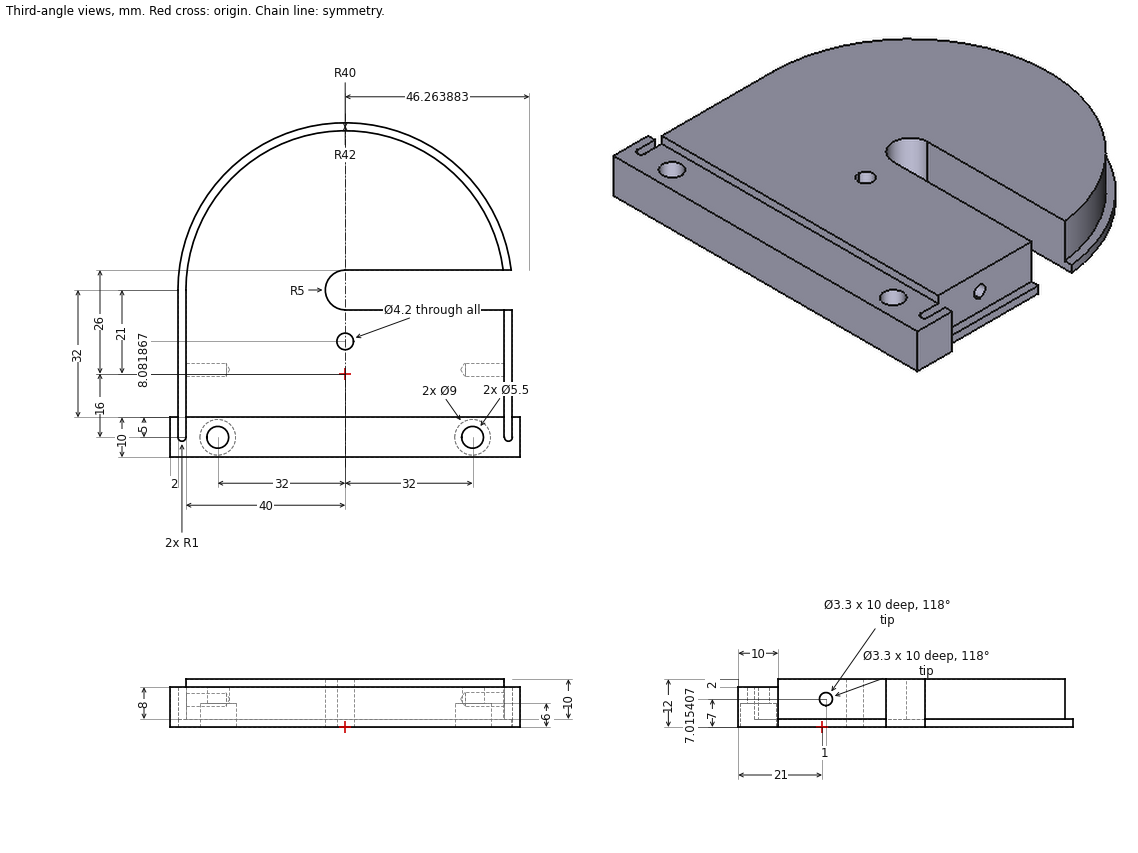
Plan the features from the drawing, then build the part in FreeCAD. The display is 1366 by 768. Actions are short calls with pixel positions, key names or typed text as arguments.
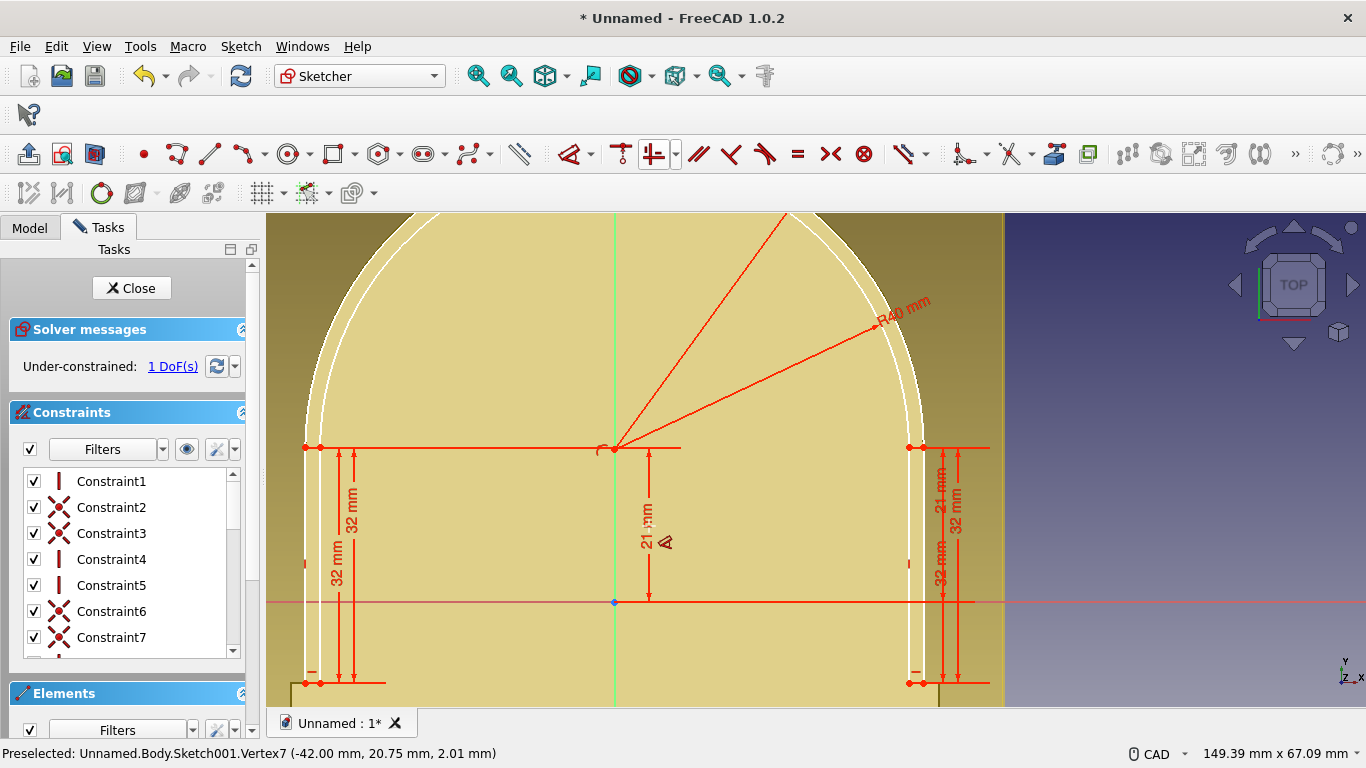
click(615, 450)
click(649, 491)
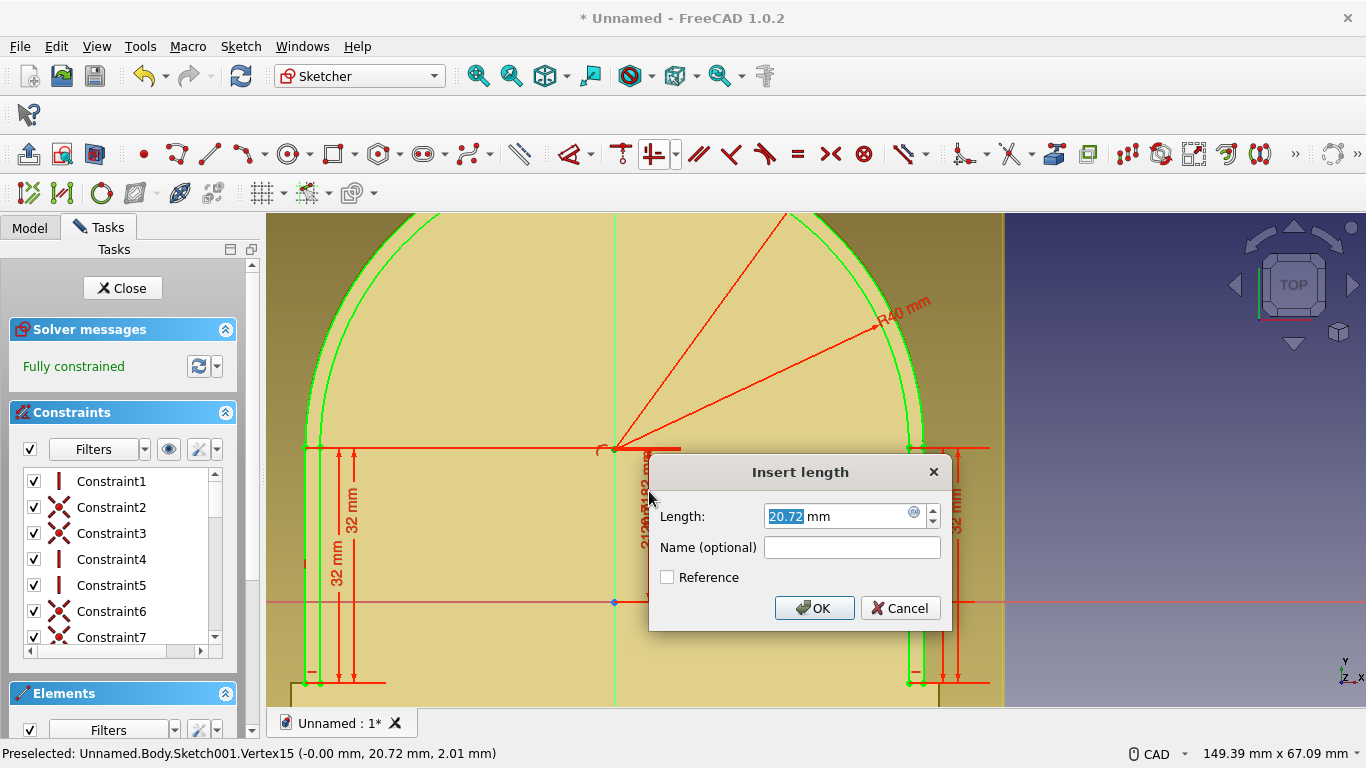
text(21)
key(Return)
key(Escape)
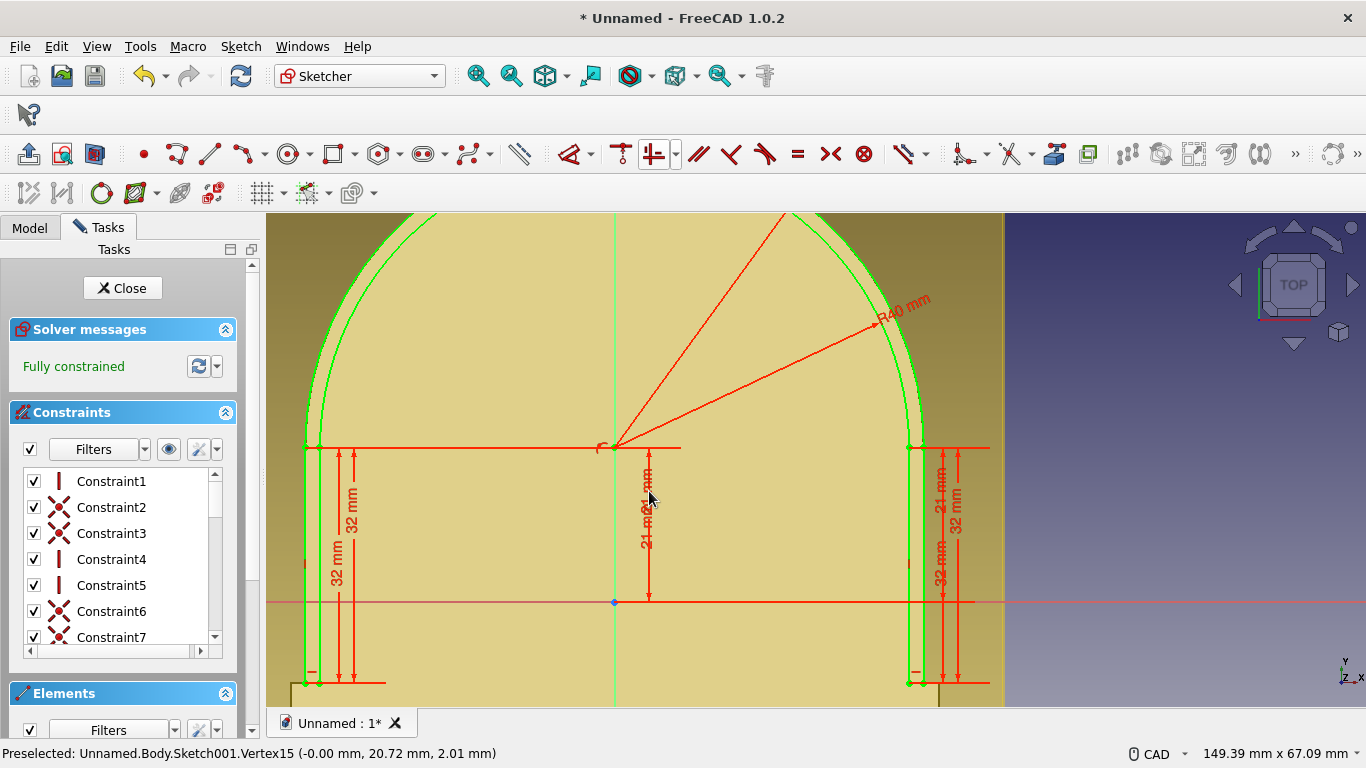
click(123, 288)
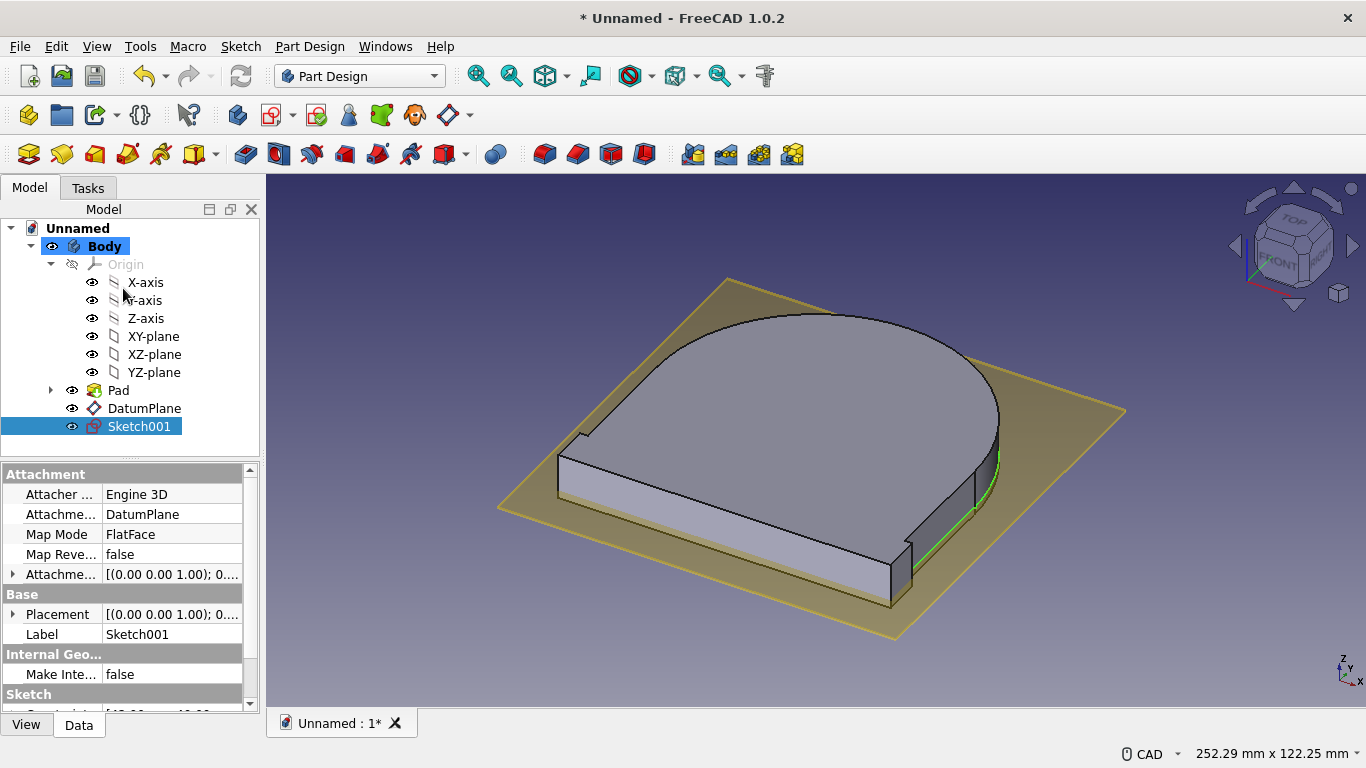
click(246, 154)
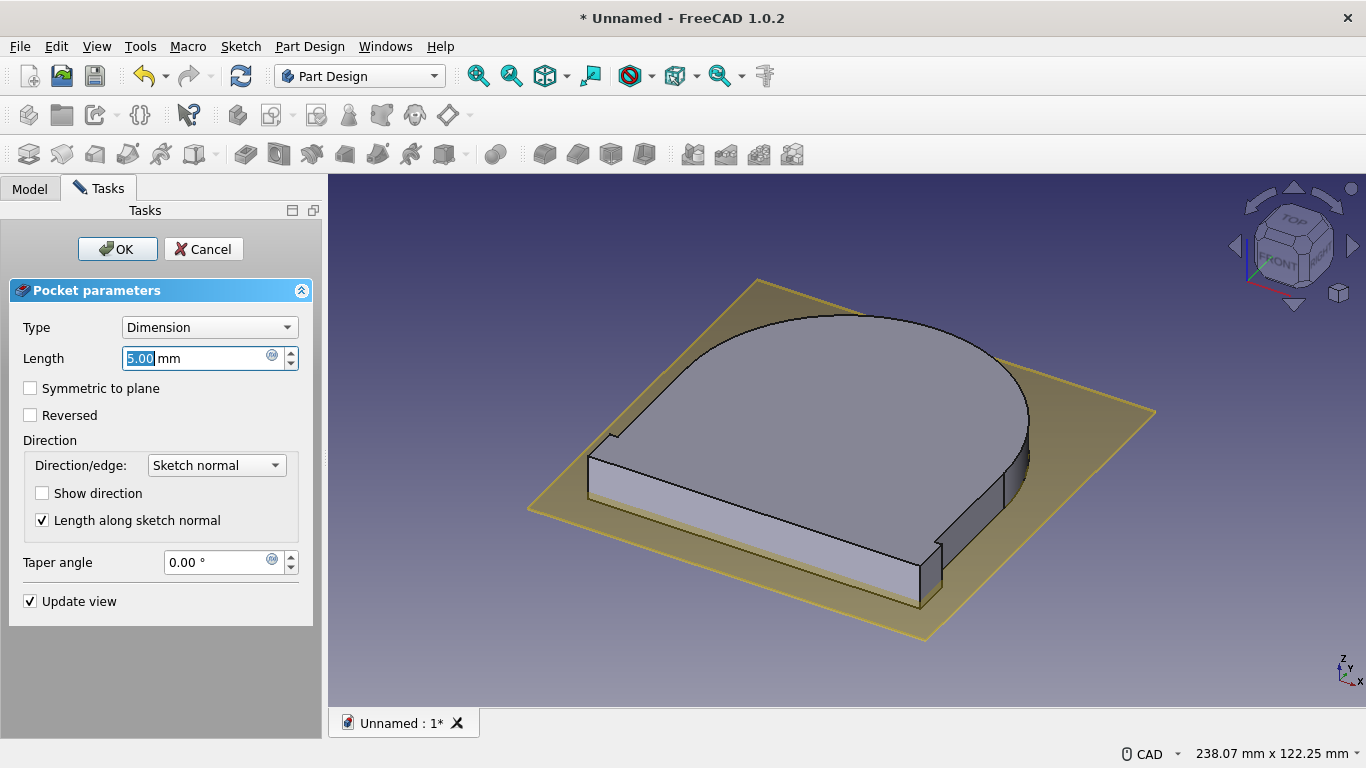
text(10)
key(Tab)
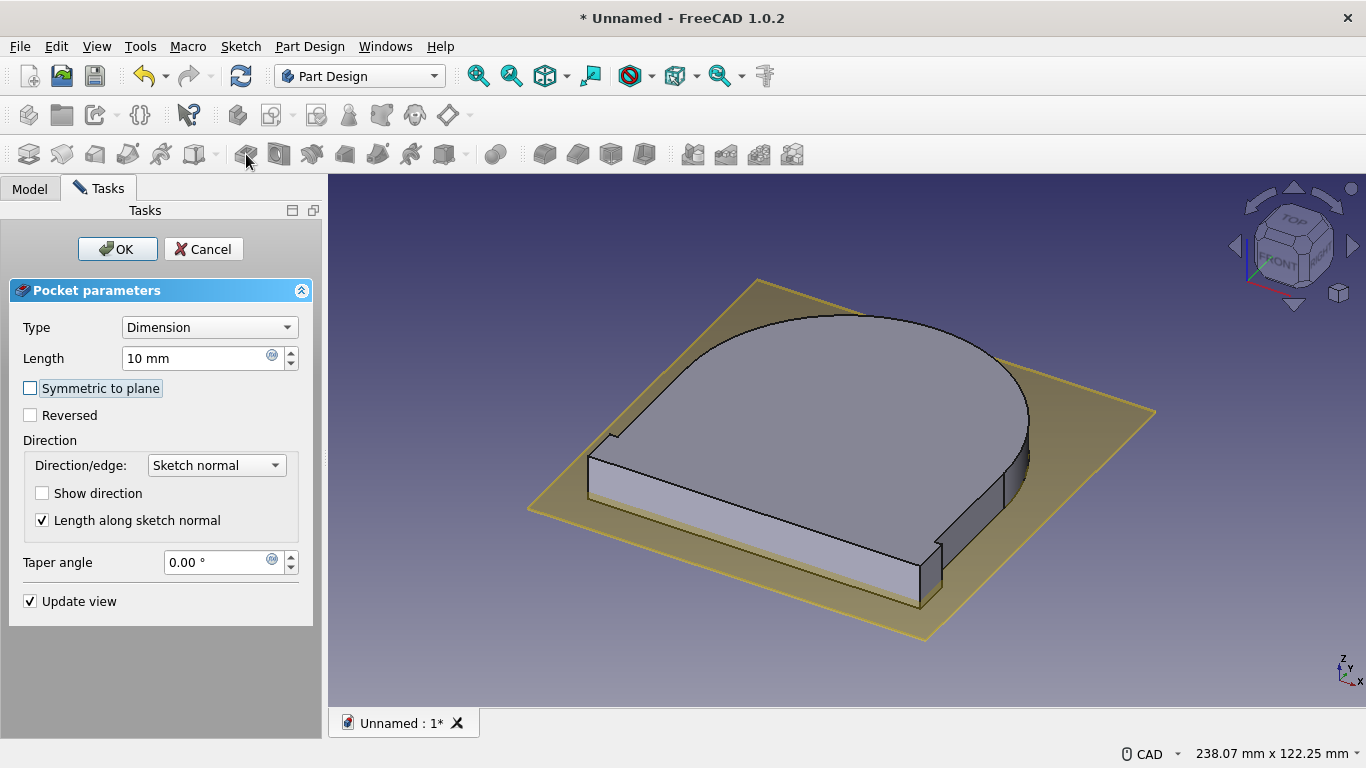
click(31, 415)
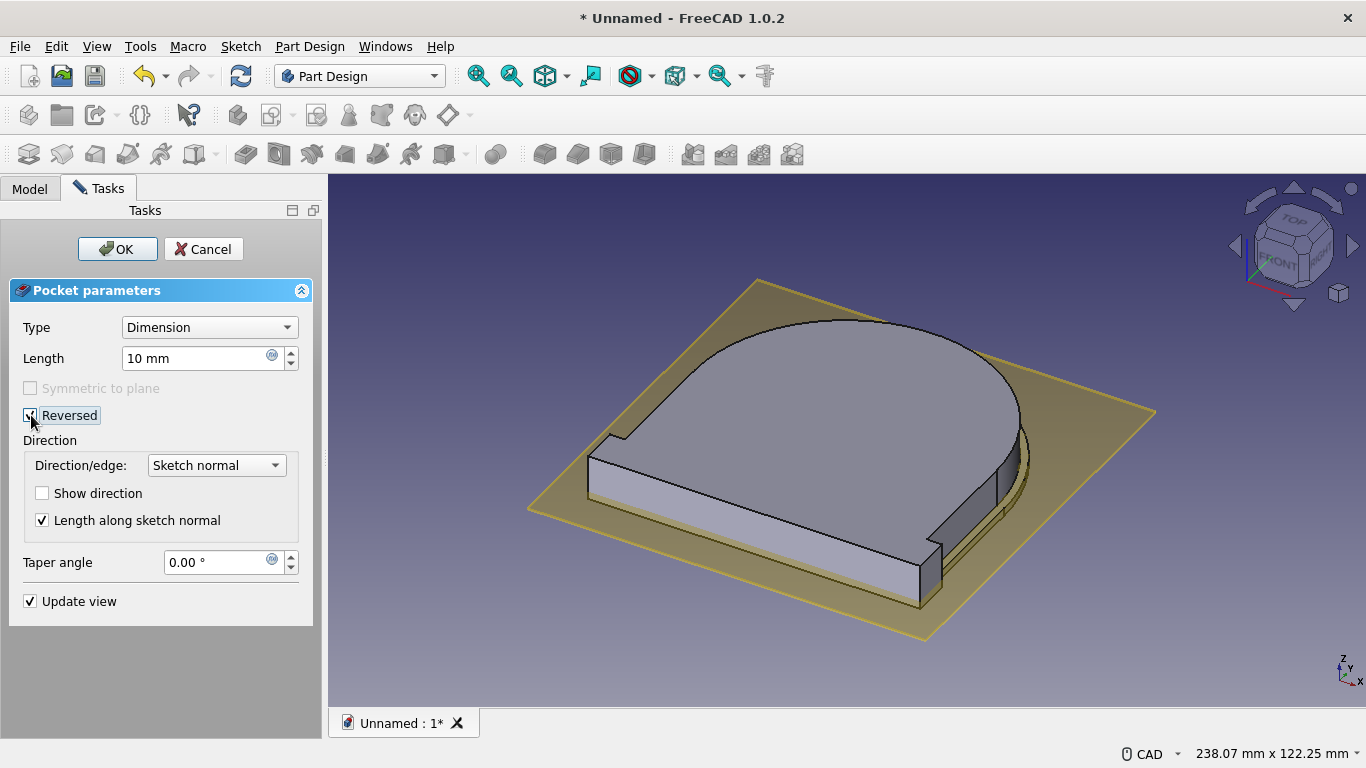
click(118, 249)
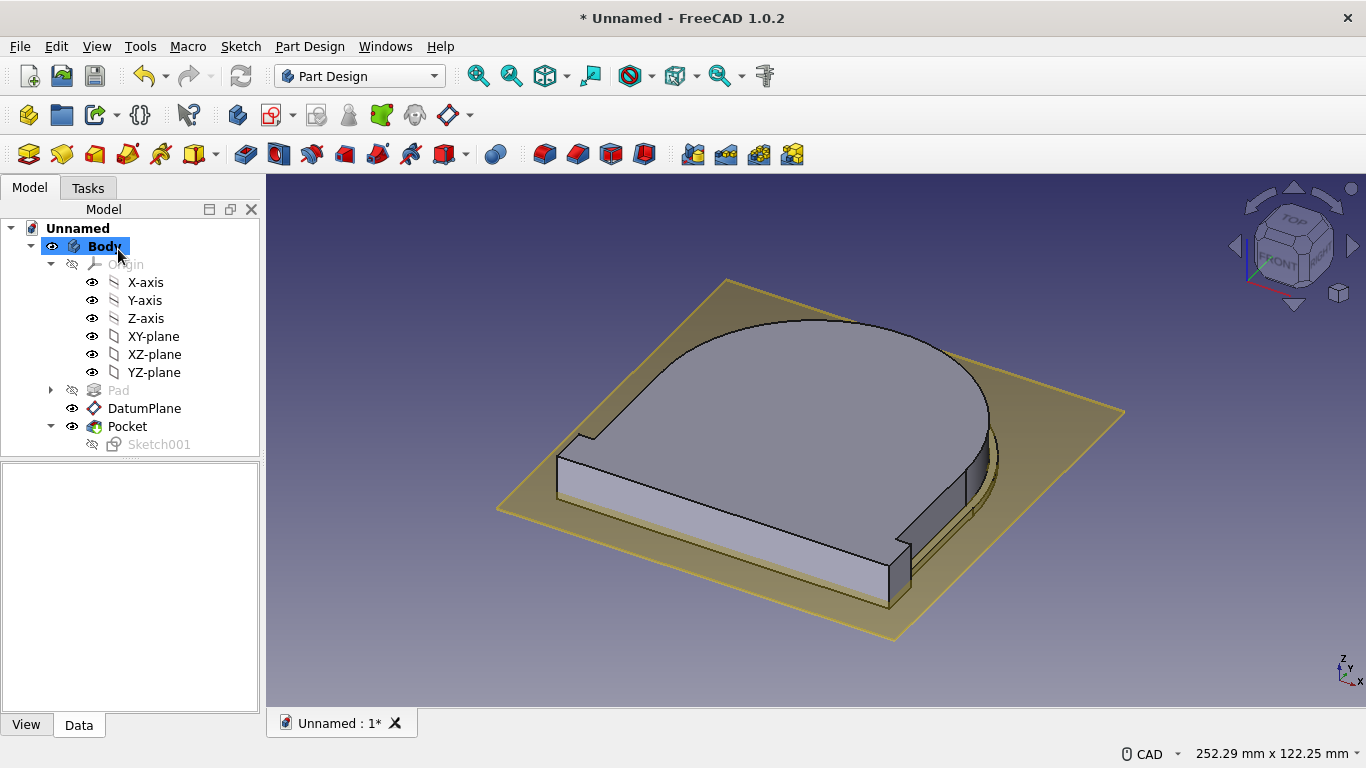
click(117, 408)
key(space)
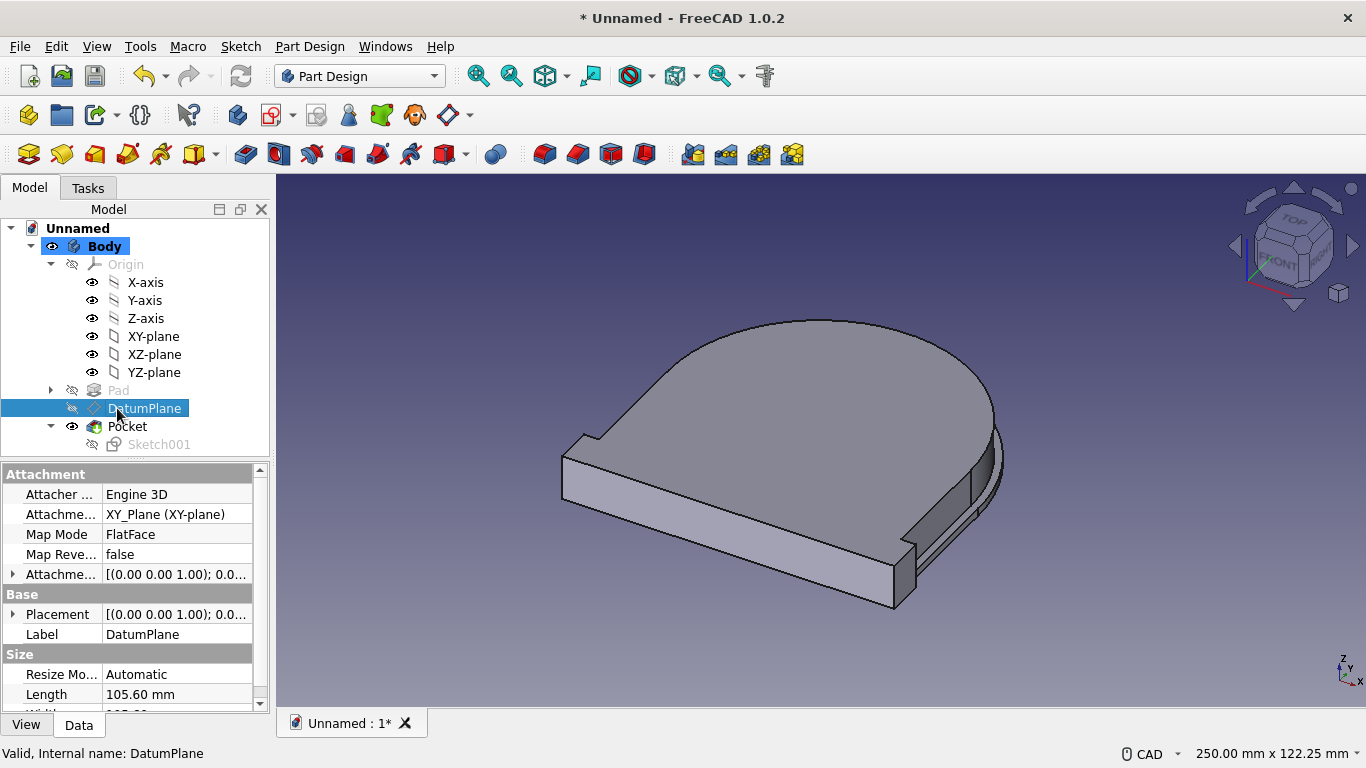
click(905, 576)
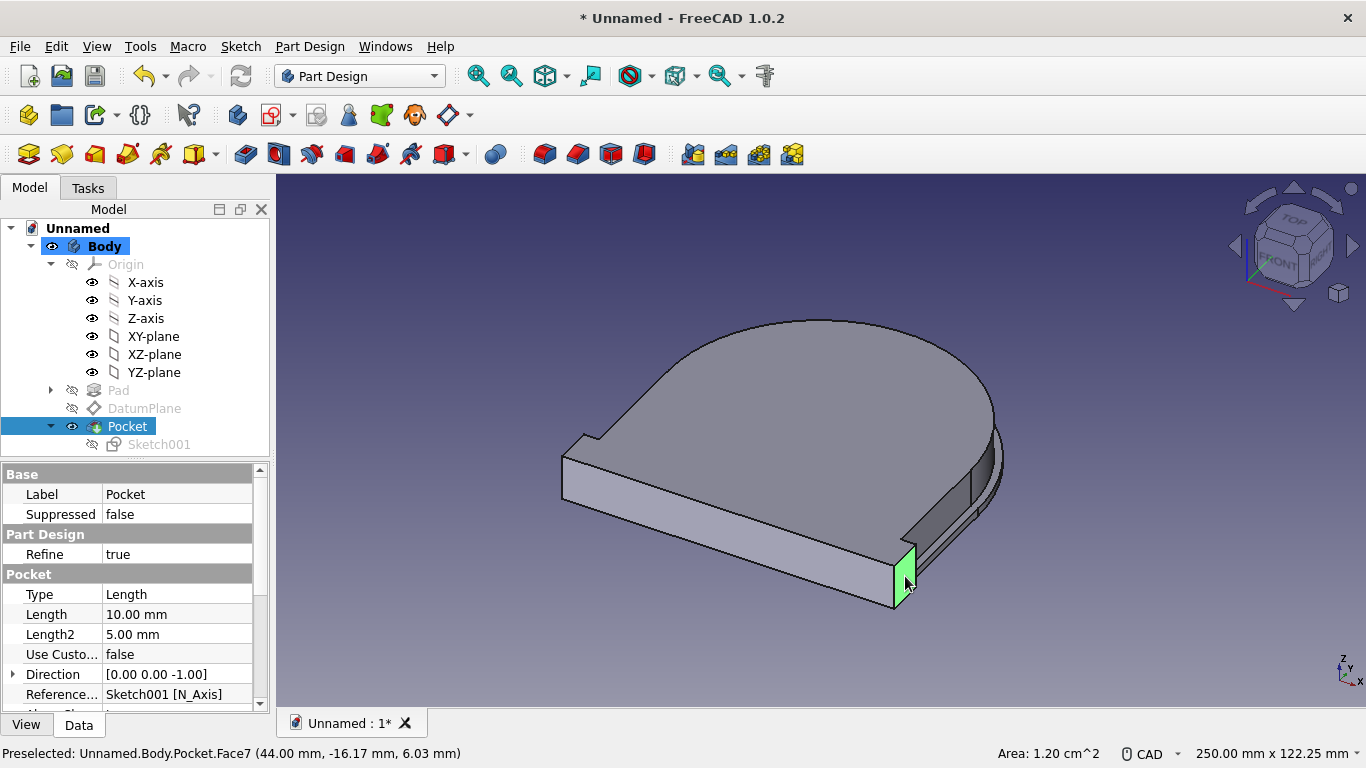
click(270, 116)